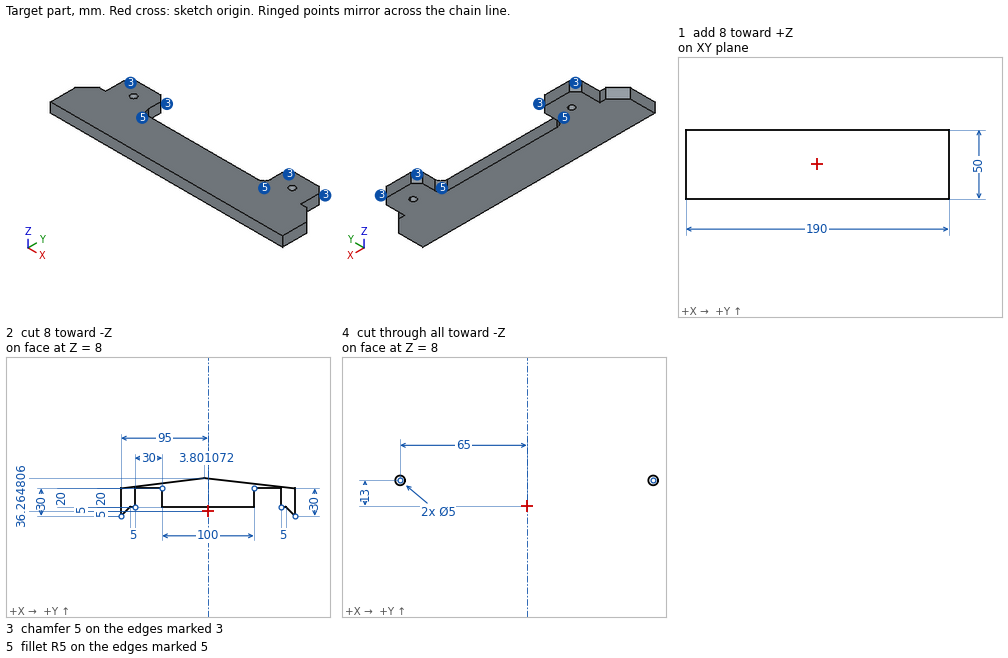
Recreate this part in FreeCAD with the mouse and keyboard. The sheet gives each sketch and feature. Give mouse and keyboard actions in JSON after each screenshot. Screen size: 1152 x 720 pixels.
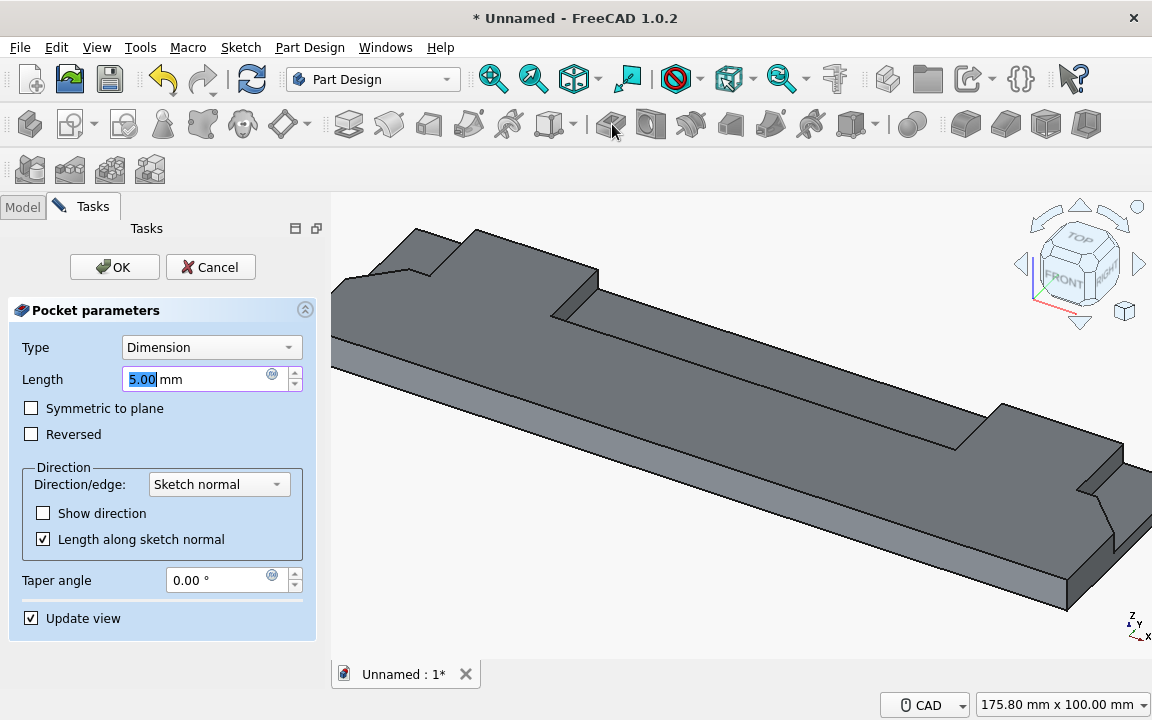
{"action": "type", "text": "8"}
{"action": "key", "text": "Tab"}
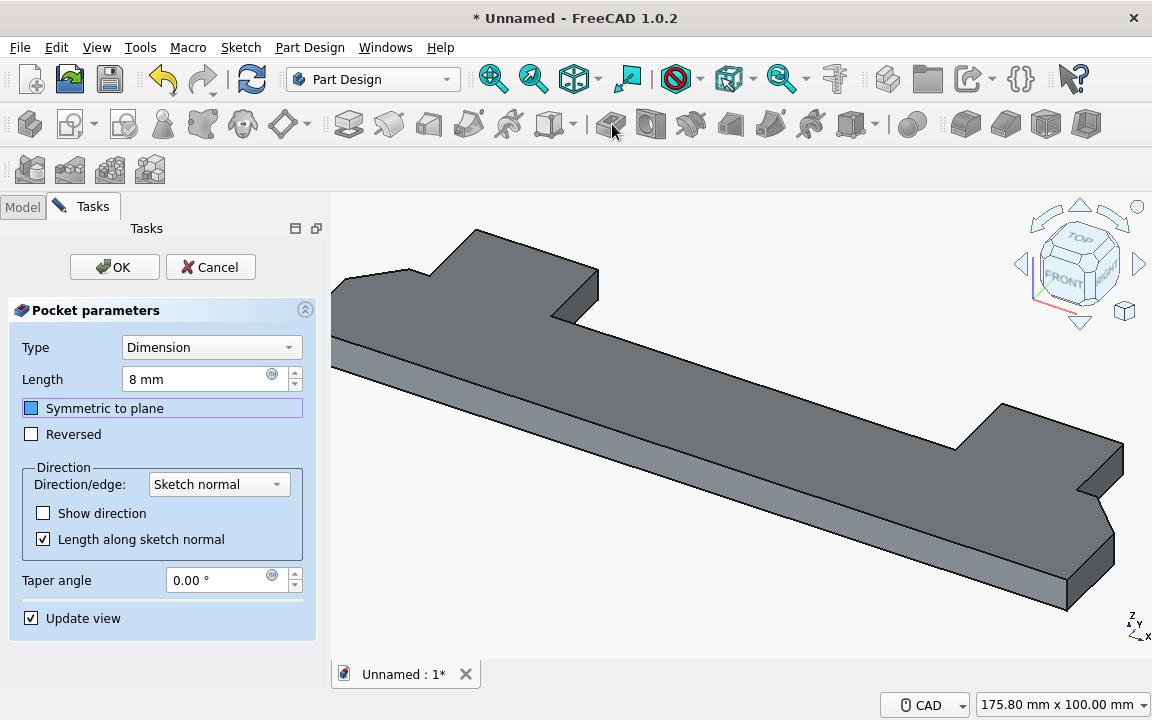
{"action": "left_click", "coordinate": [115, 267]}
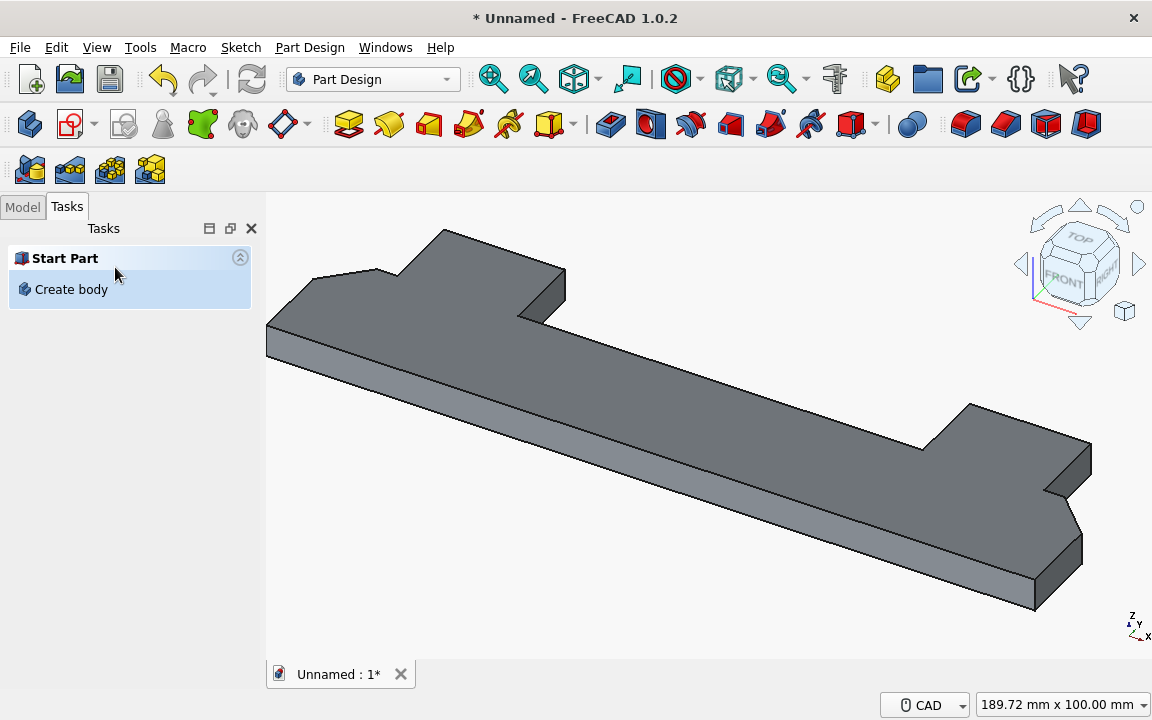
{"action": "key", "text": "0"}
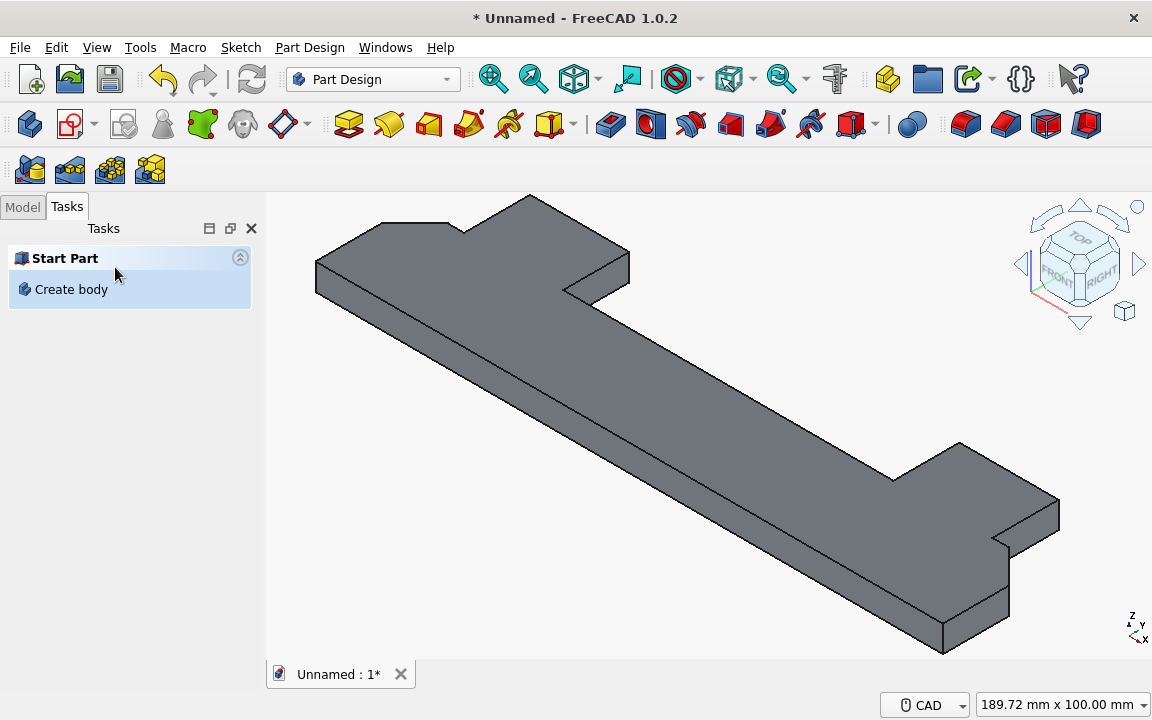
{"action": "left_click", "coordinate": [494, 80]}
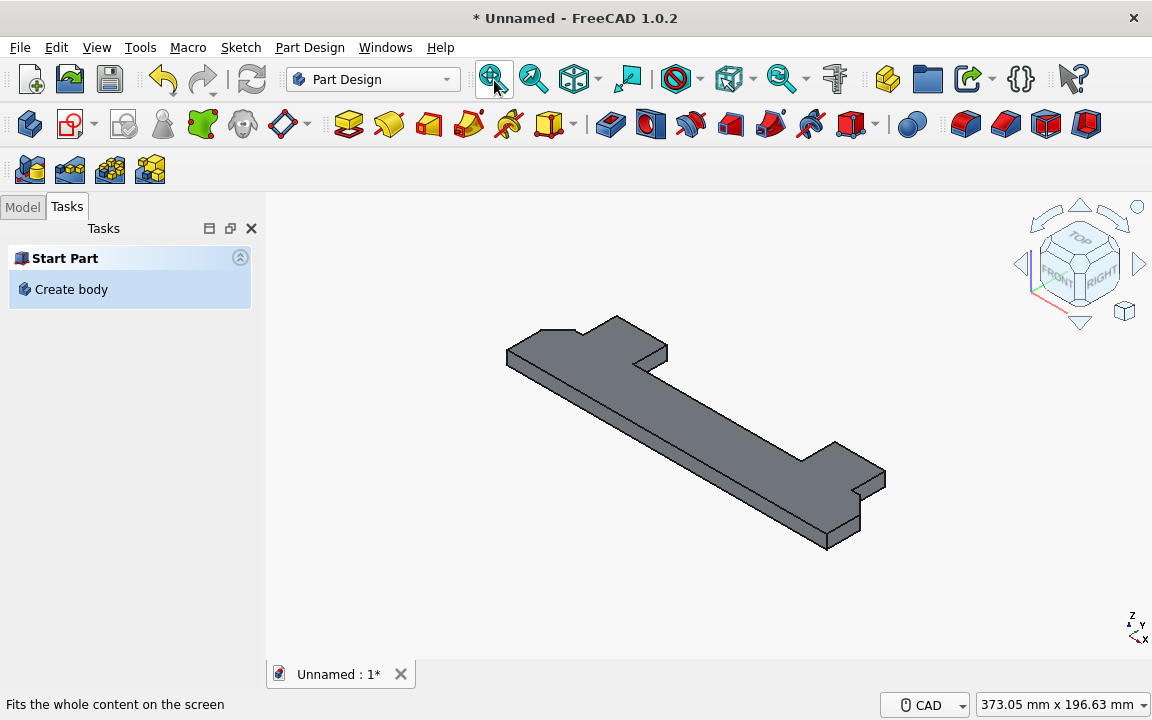
{"action": "scroll", "coordinate": [885, 478], "scroll_direction": "up", "scroll_amount": 4}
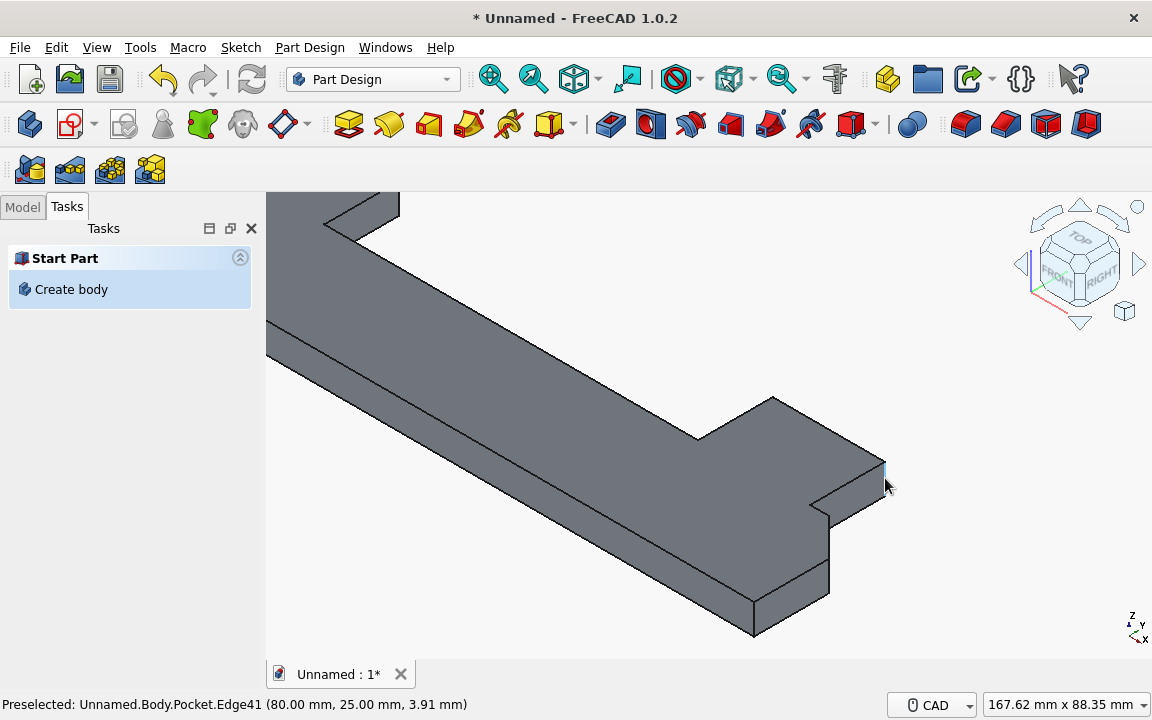
{"action": "left_click", "coordinate": [494, 80]}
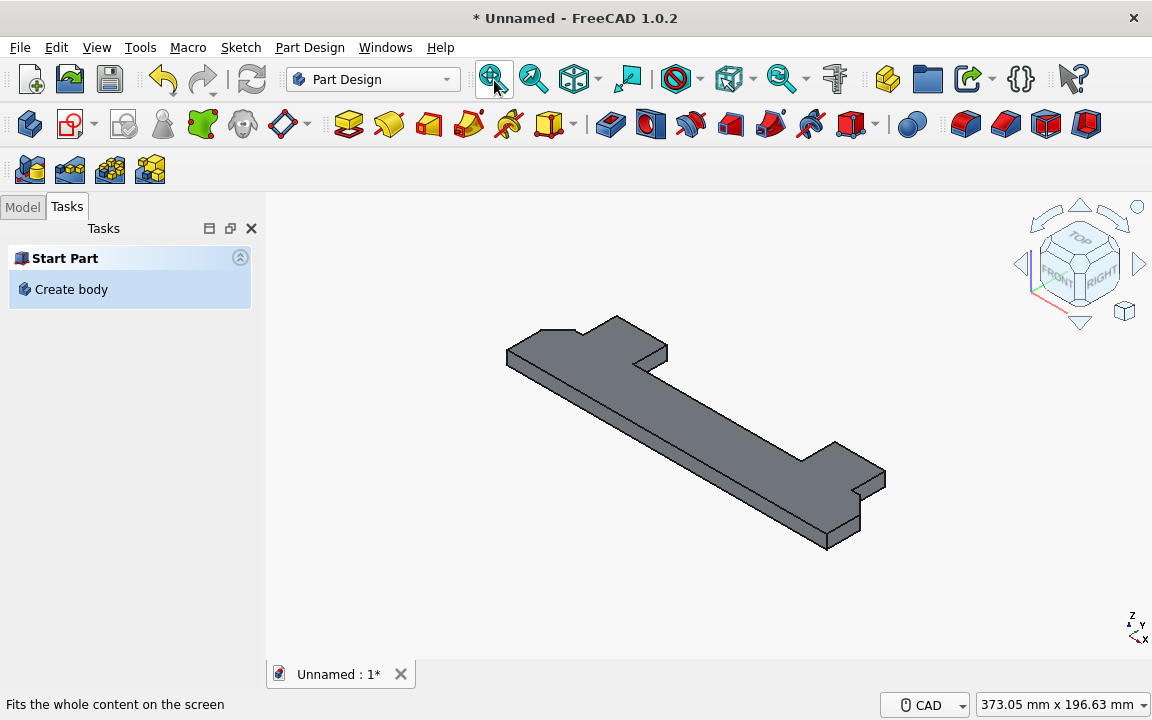
{"action": "key", "text": "2"}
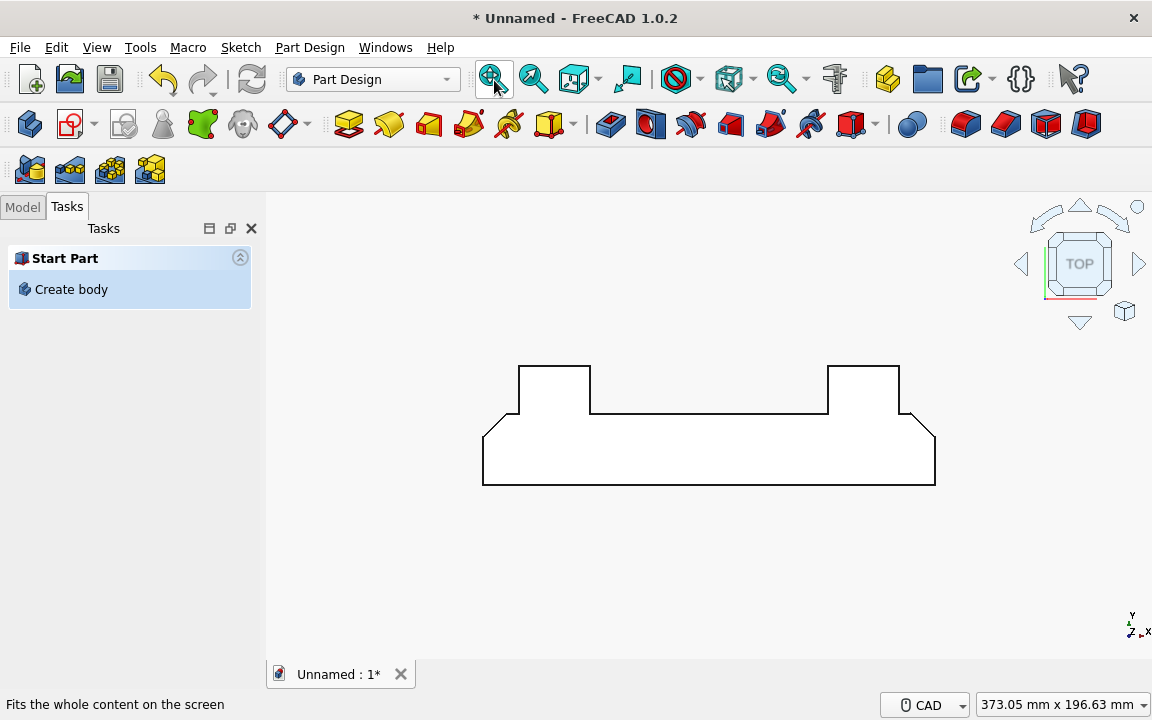
{"action": "scroll", "coordinate": [899, 365], "scroll_direction": "up", "scroll_amount": 4}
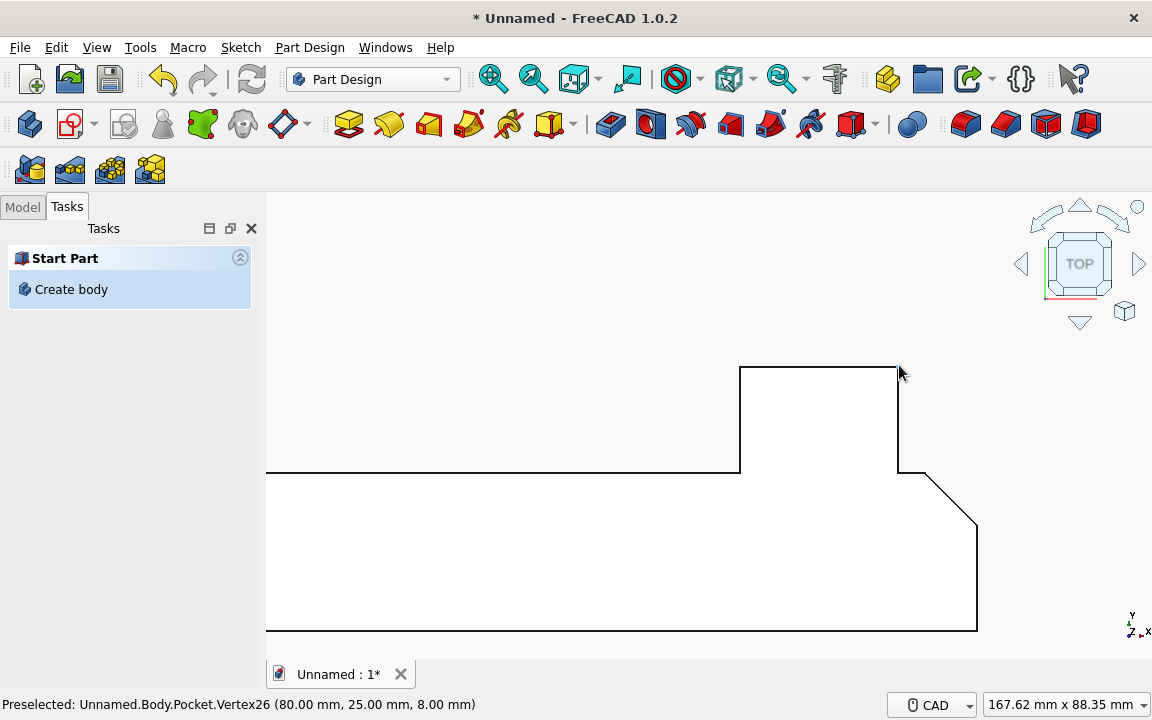
{"action": "left_click", "coordinate": [494, 80]}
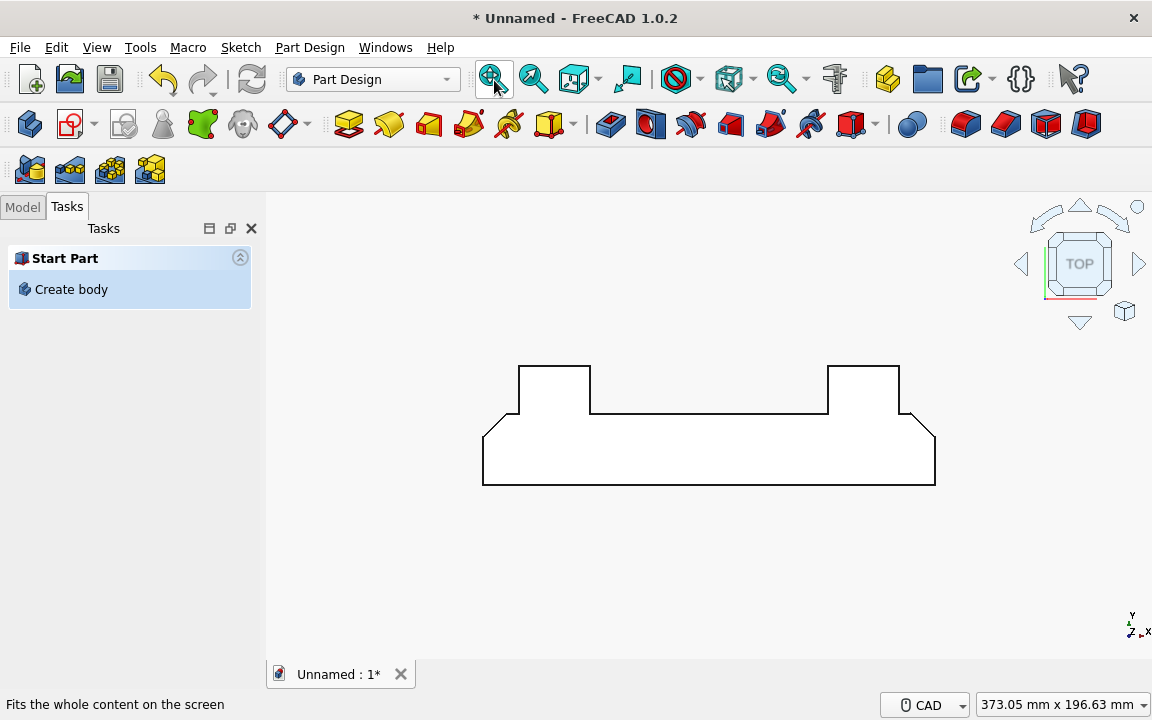
{"action": "key", "text": "1"}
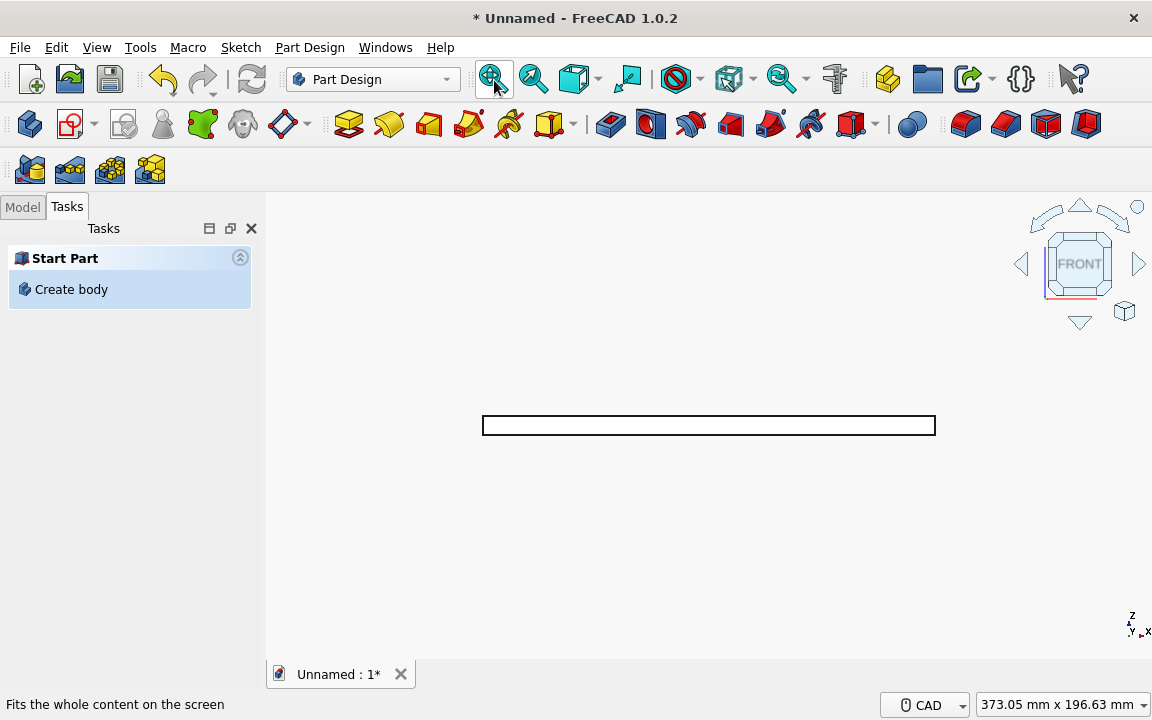
{"action": "scroll", "coordinate": [899, 424], "scroll_direction": "up", "scroll_amount": 4}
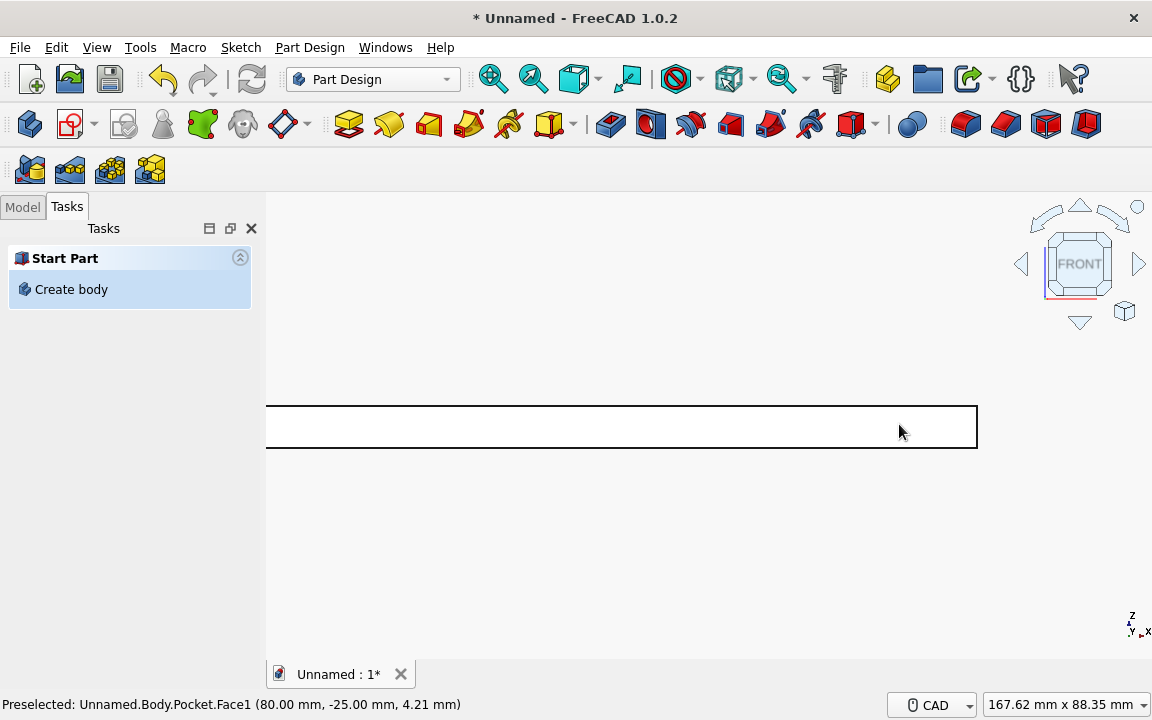
{"action": "left_click", "coordinate": [494, 80]}